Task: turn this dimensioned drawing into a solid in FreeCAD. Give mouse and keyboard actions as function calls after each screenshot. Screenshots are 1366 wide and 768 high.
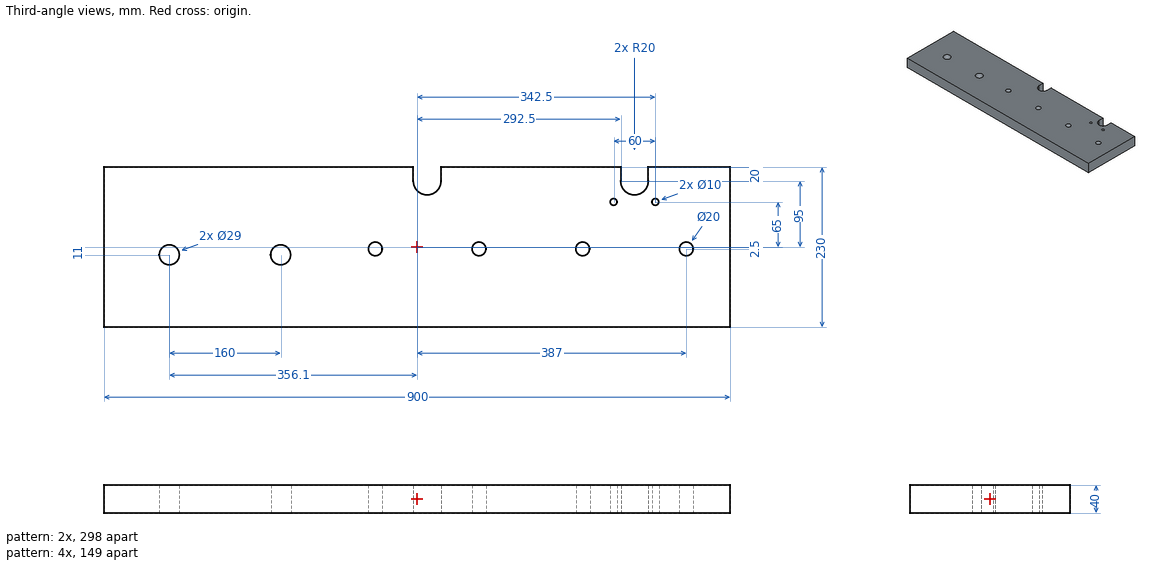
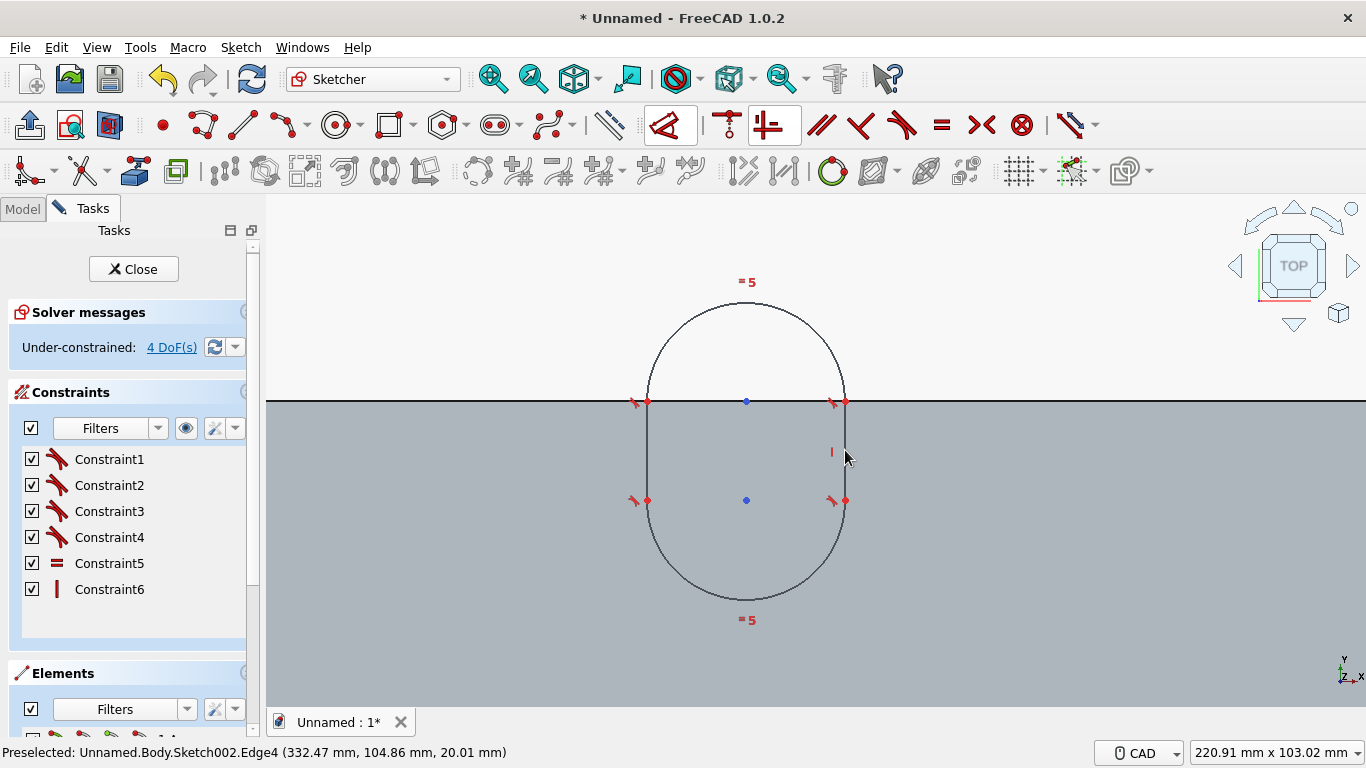
click(688, 581)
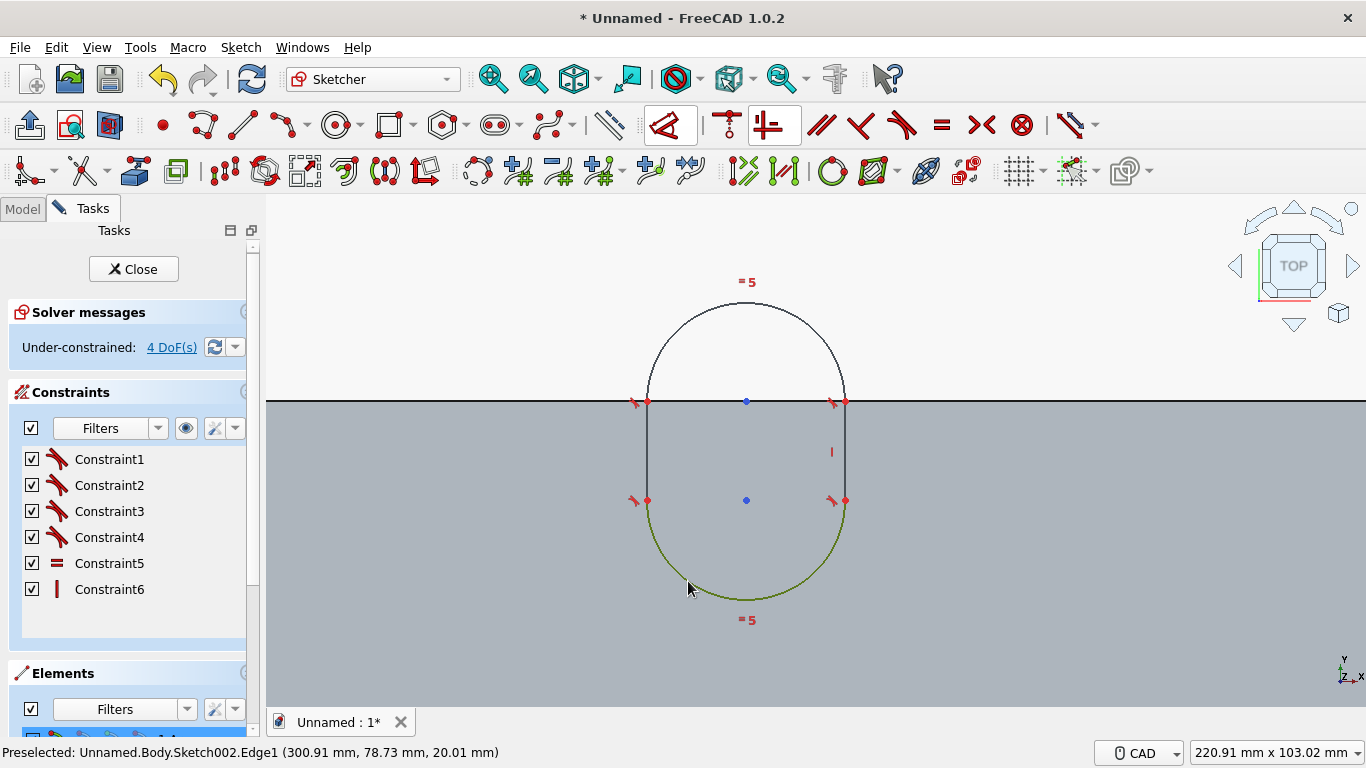
key(k)
key(r)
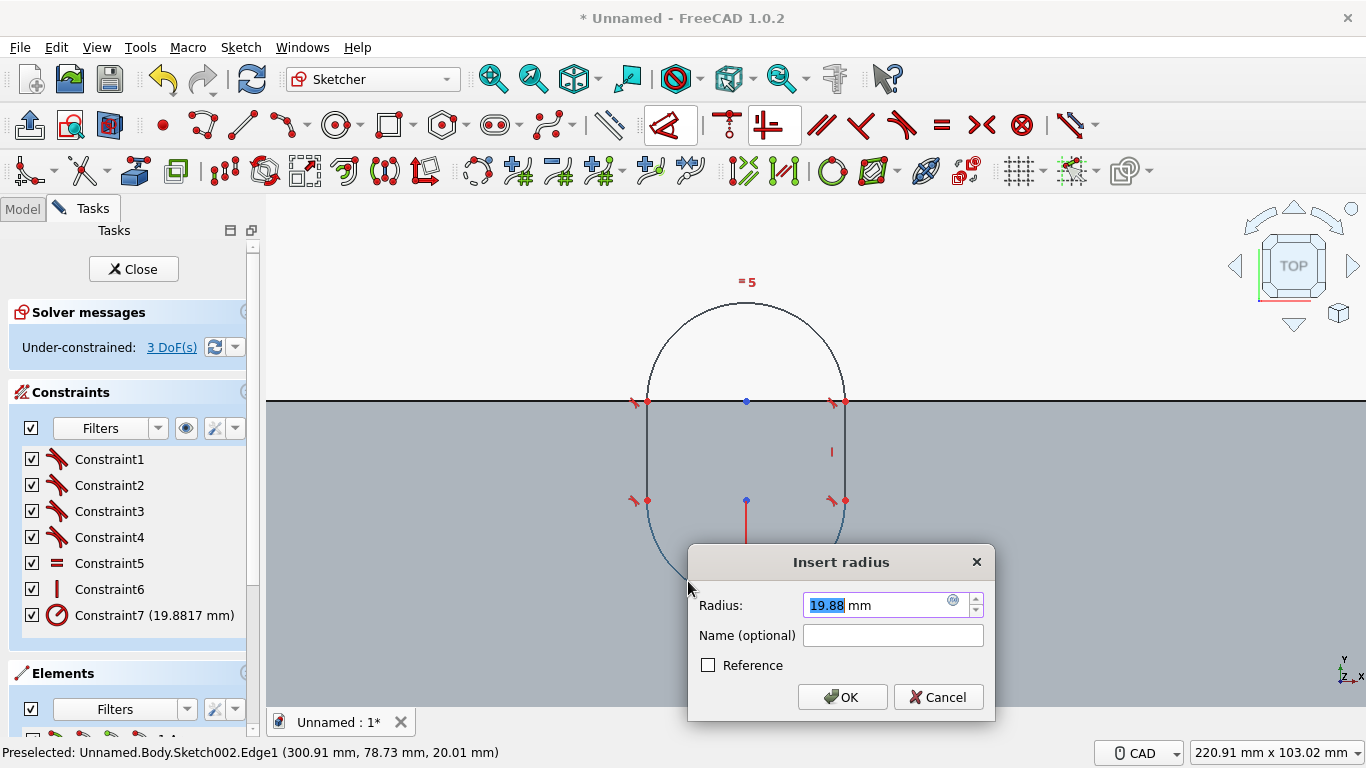
text(20)
key(Return)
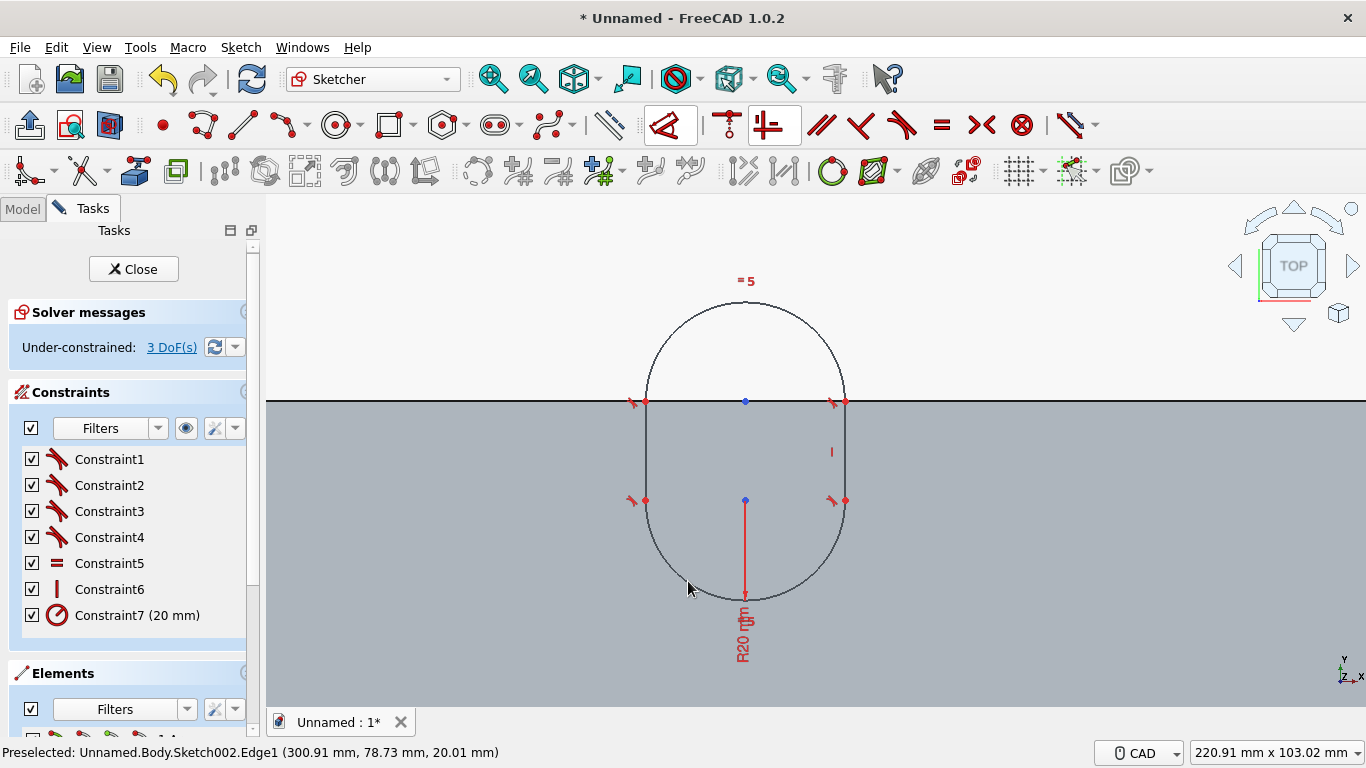
click(646, 471)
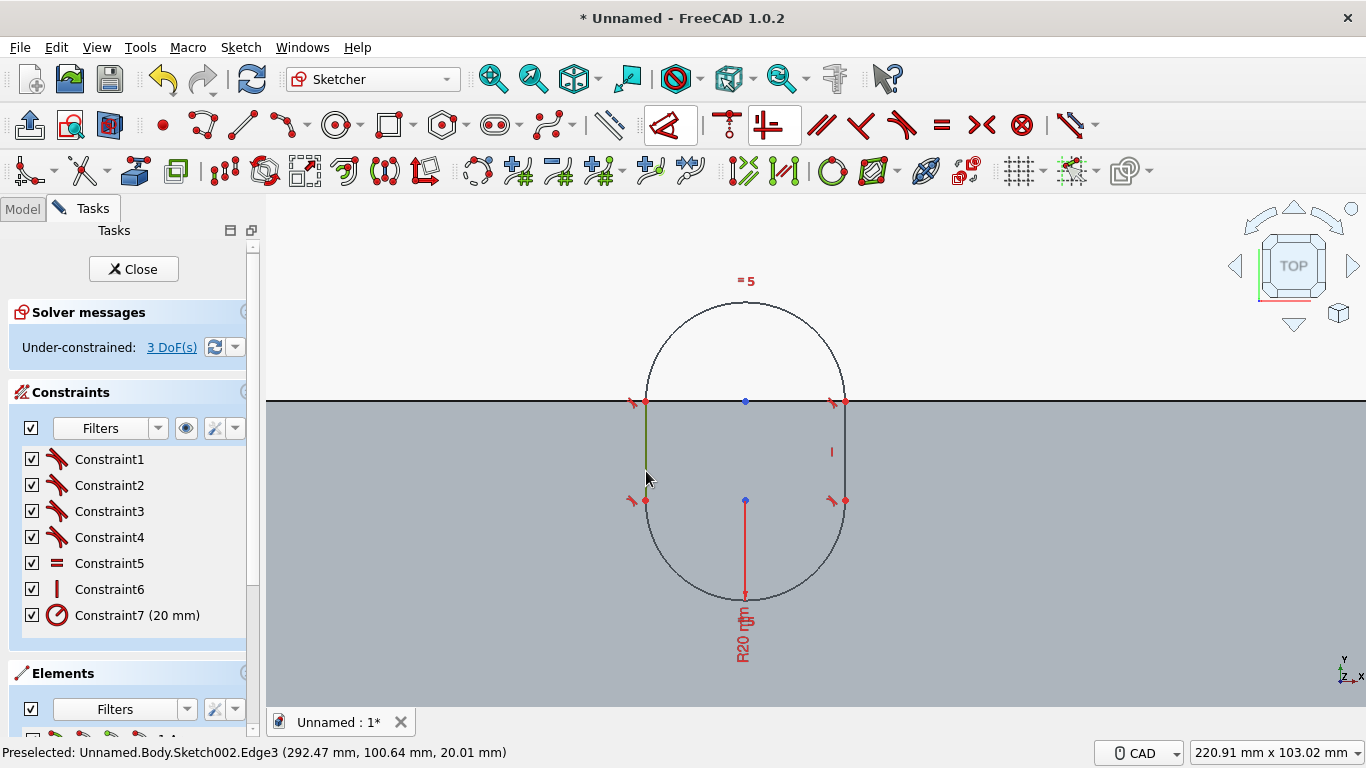
key(i)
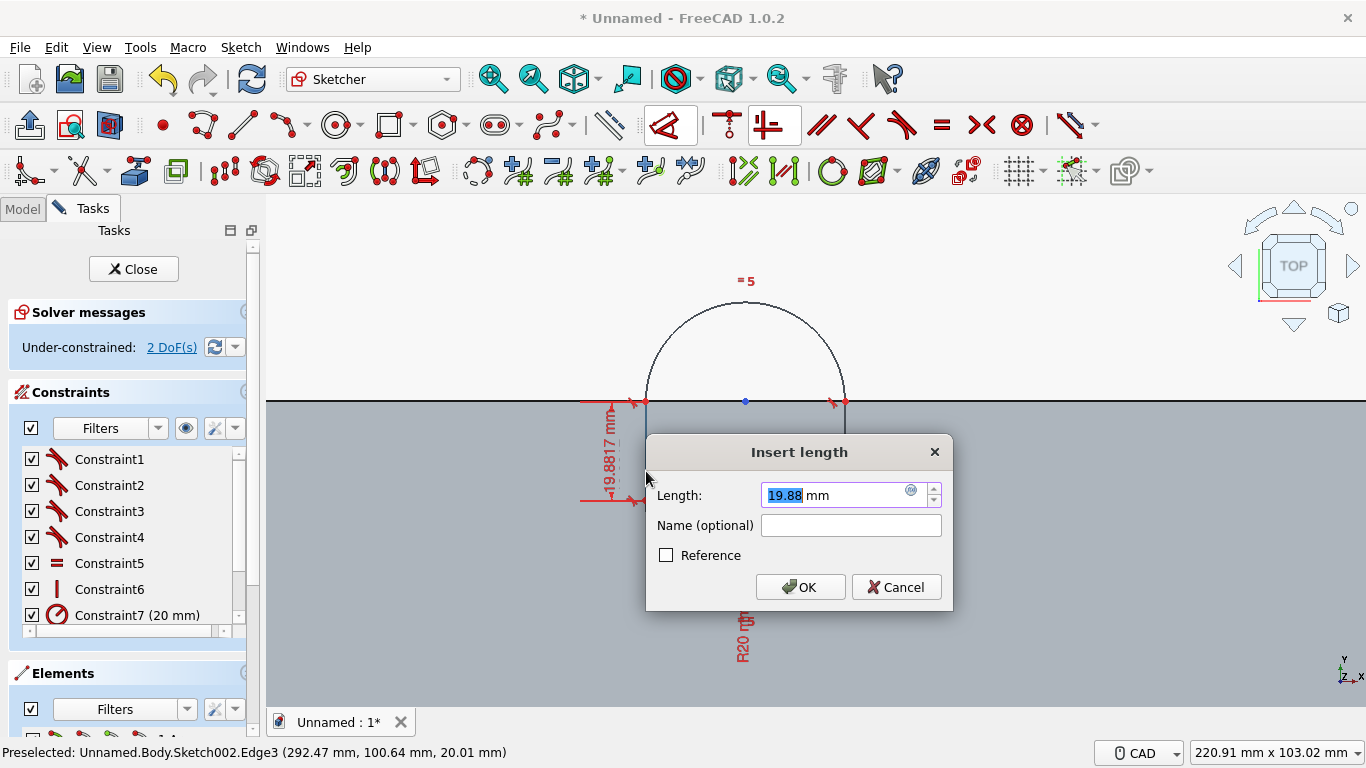
text(20)
key(Return)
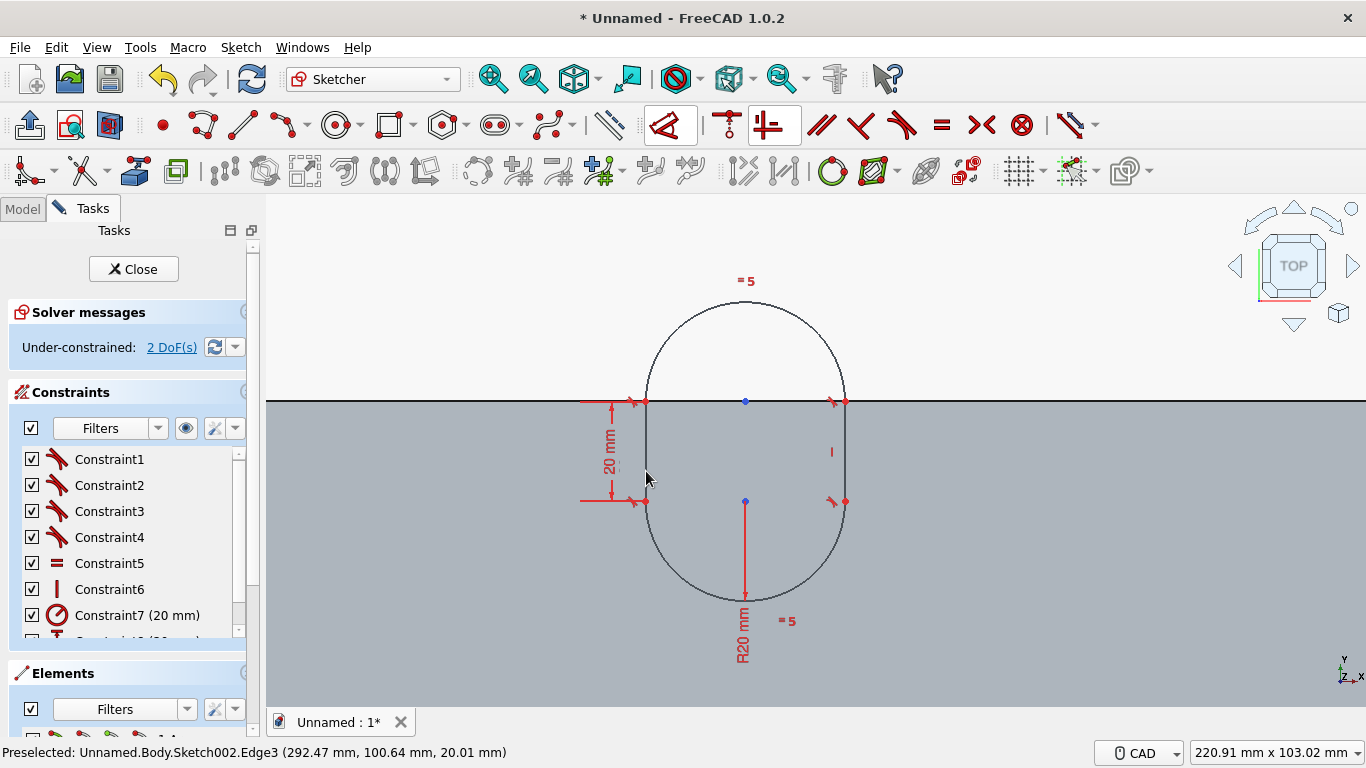
click(646, 501)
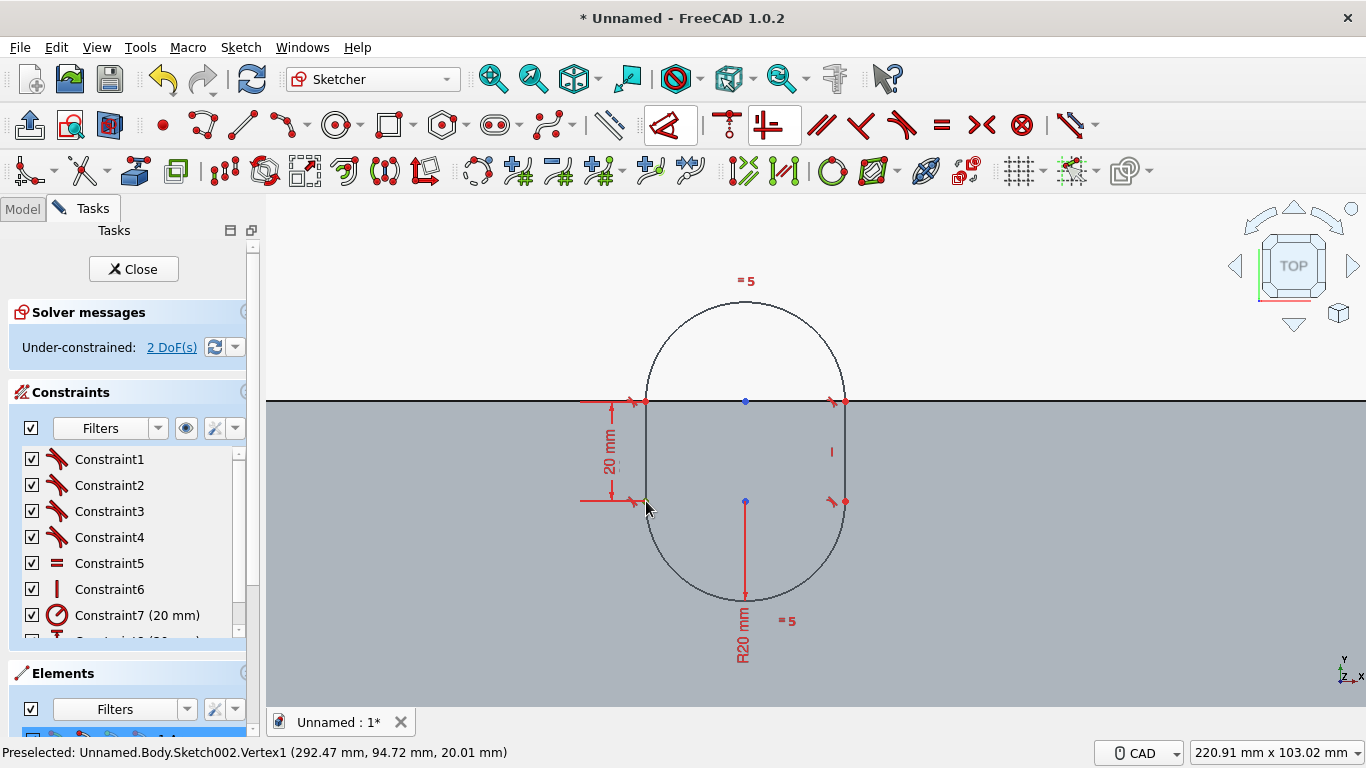
key(i)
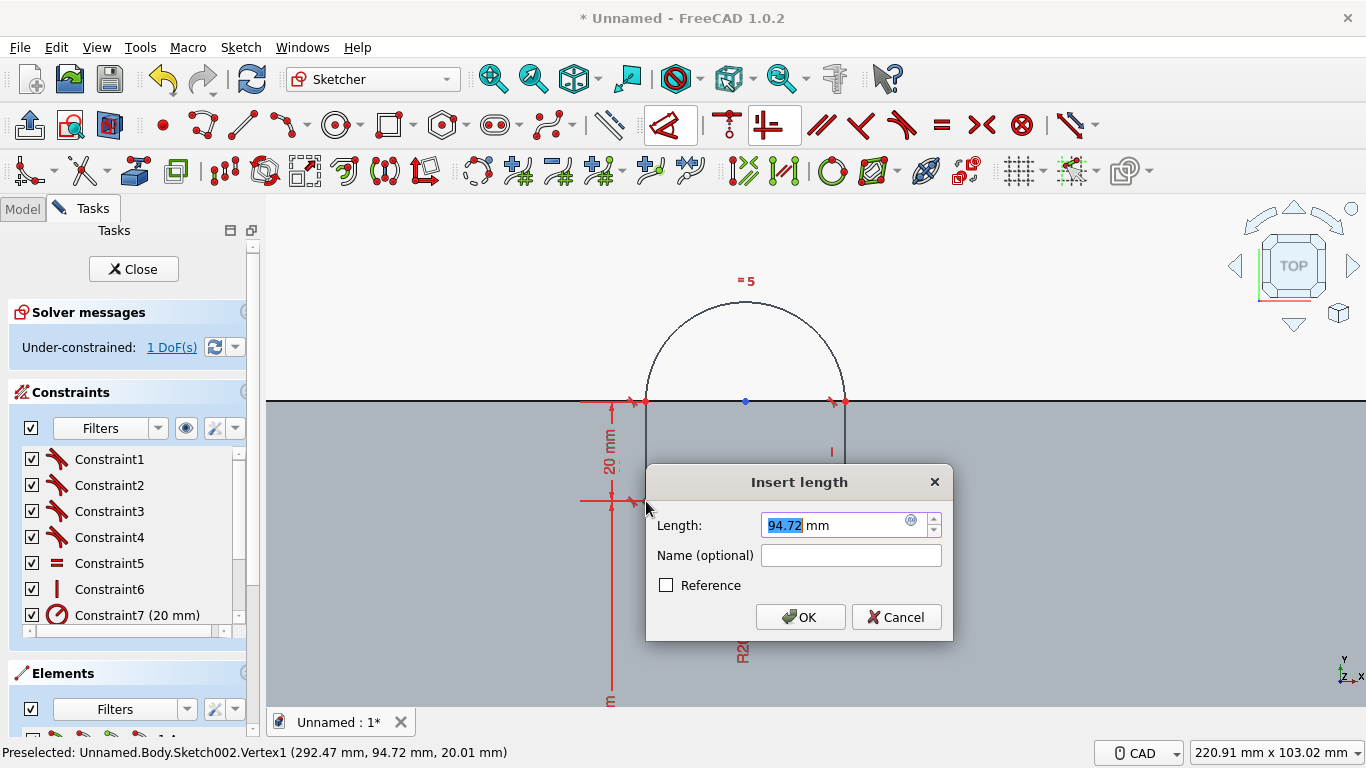
text(95)
key(Return)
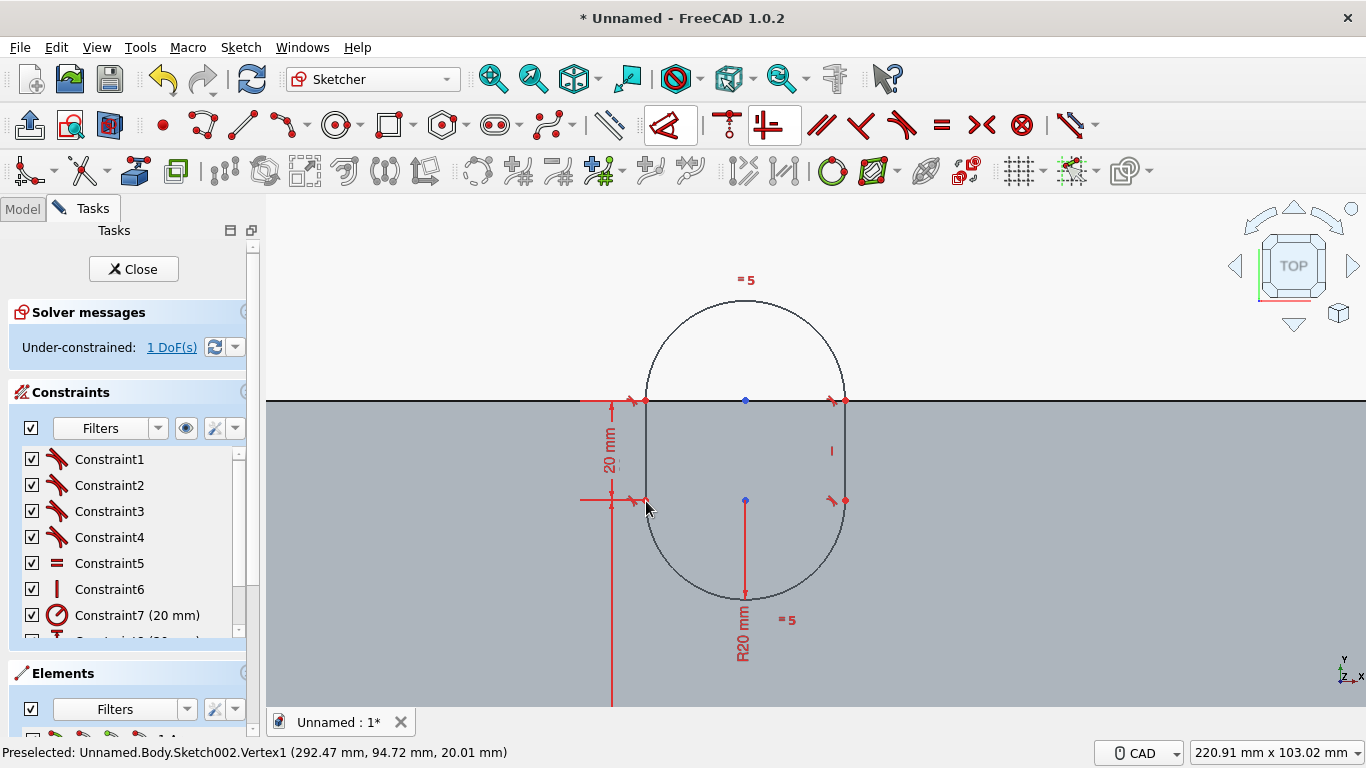
click(646, 500)